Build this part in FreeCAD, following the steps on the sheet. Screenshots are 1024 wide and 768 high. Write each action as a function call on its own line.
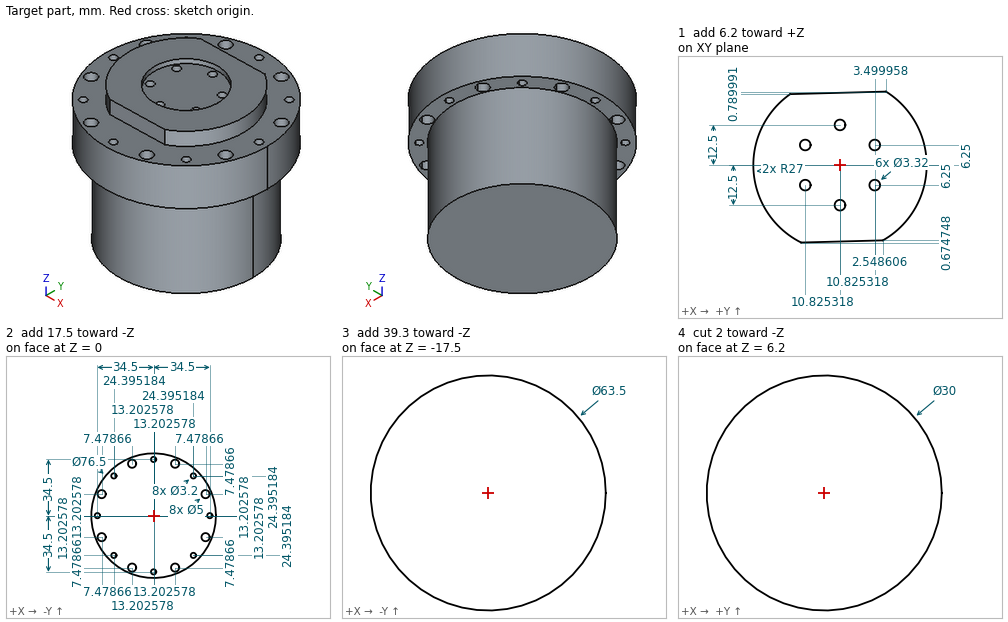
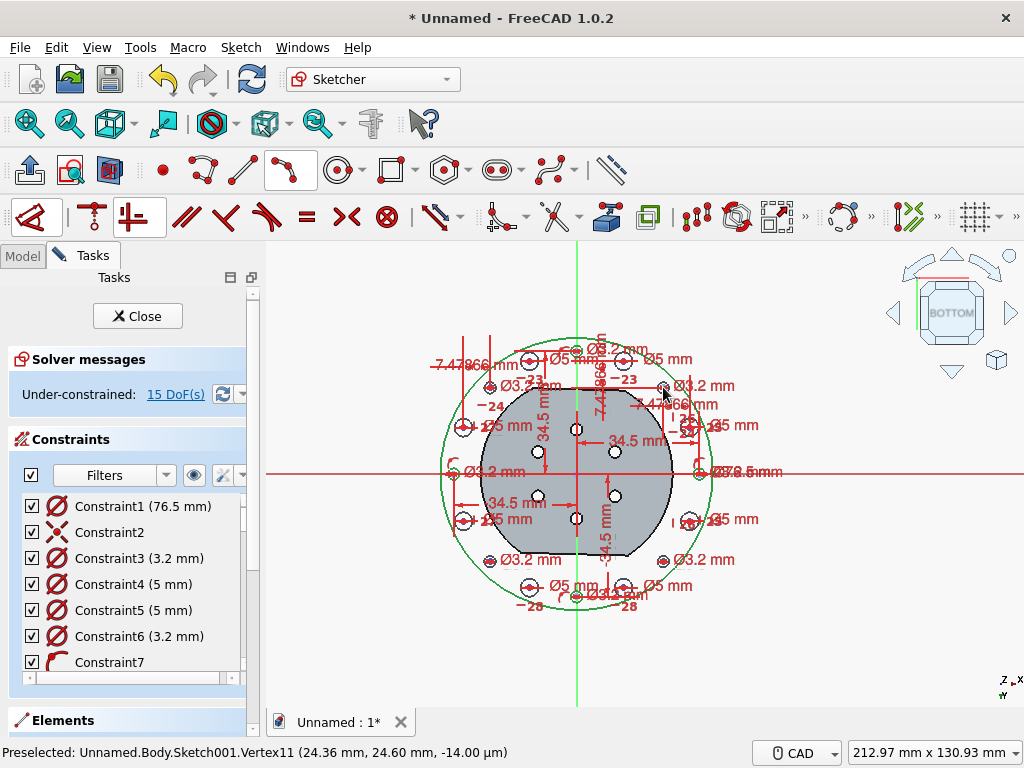
scroll(624, 588, up, 2)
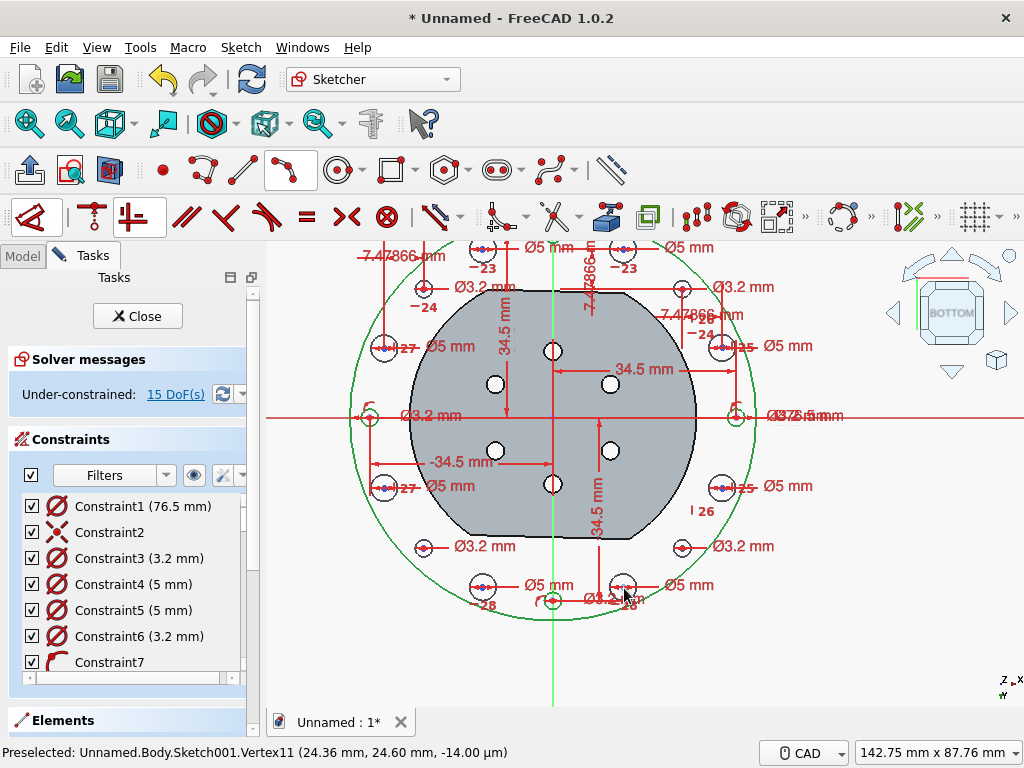
click(623, 587)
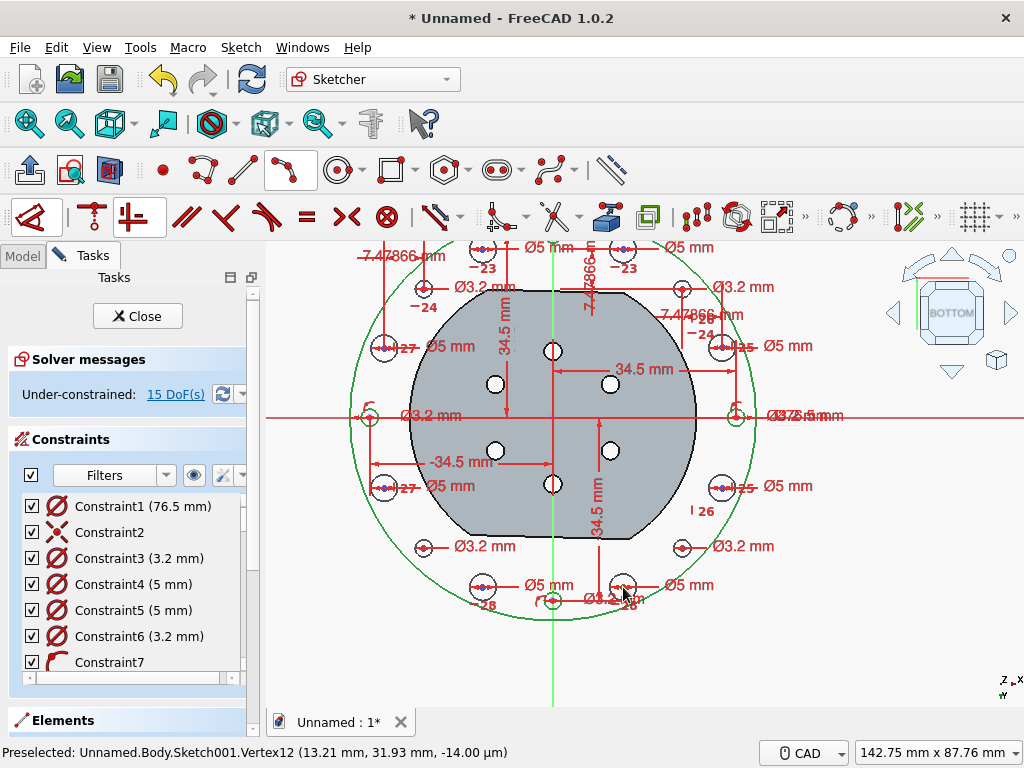
click(56, 218)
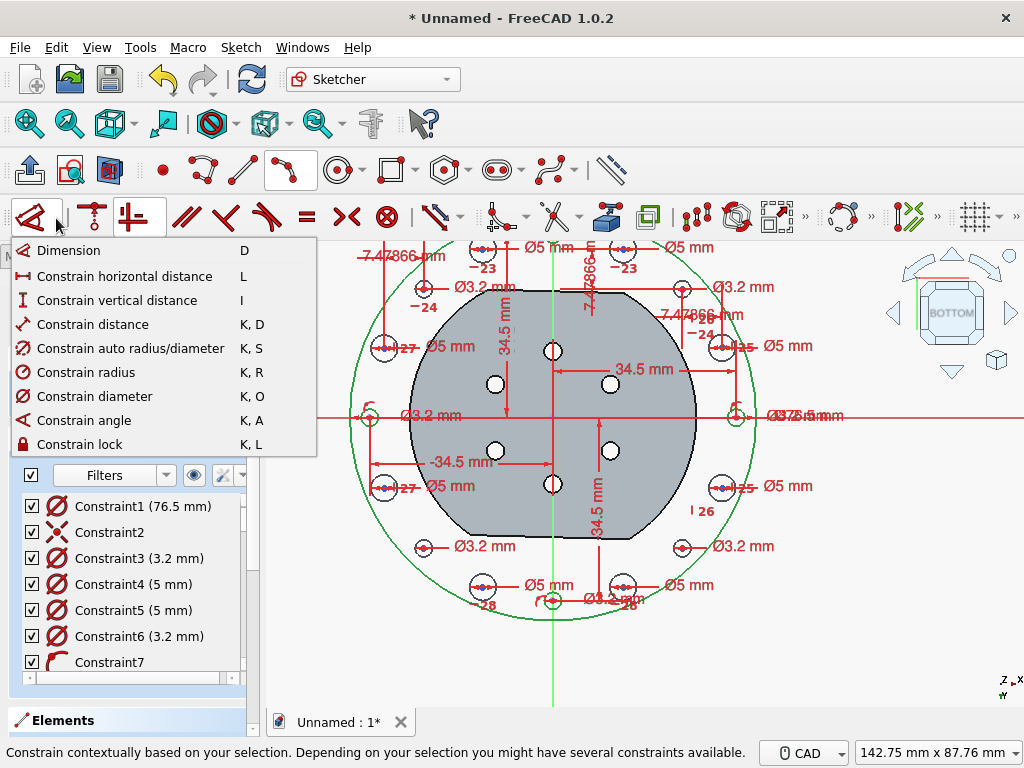
click(164, 300)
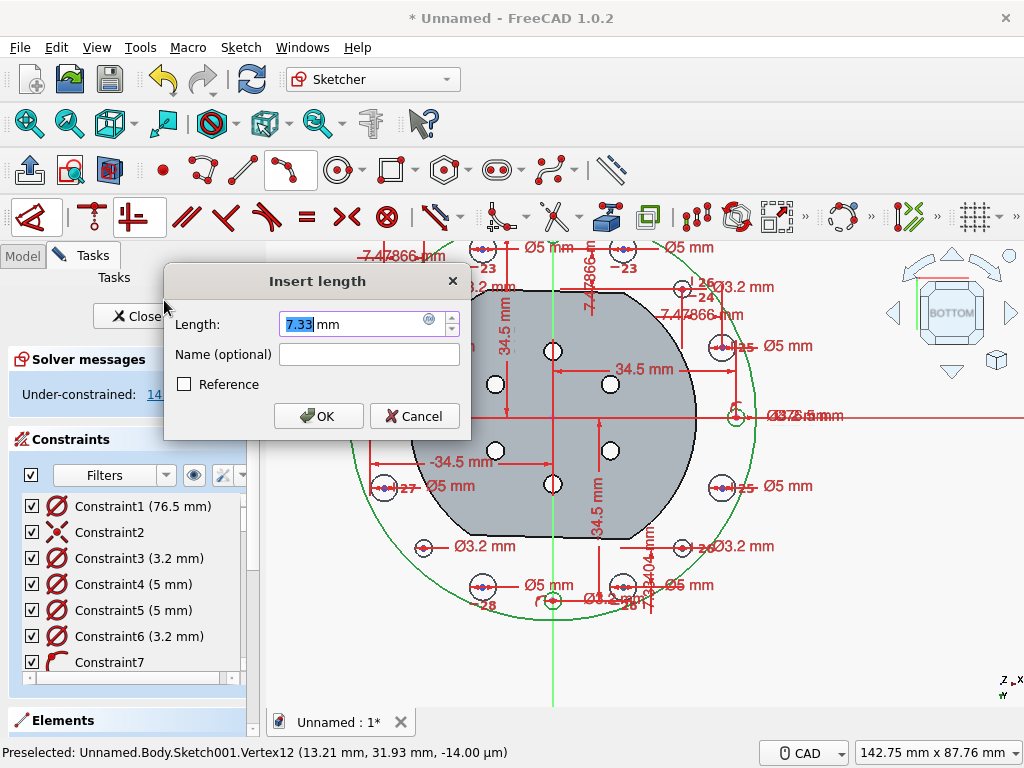
text(7.47866)
key(Return)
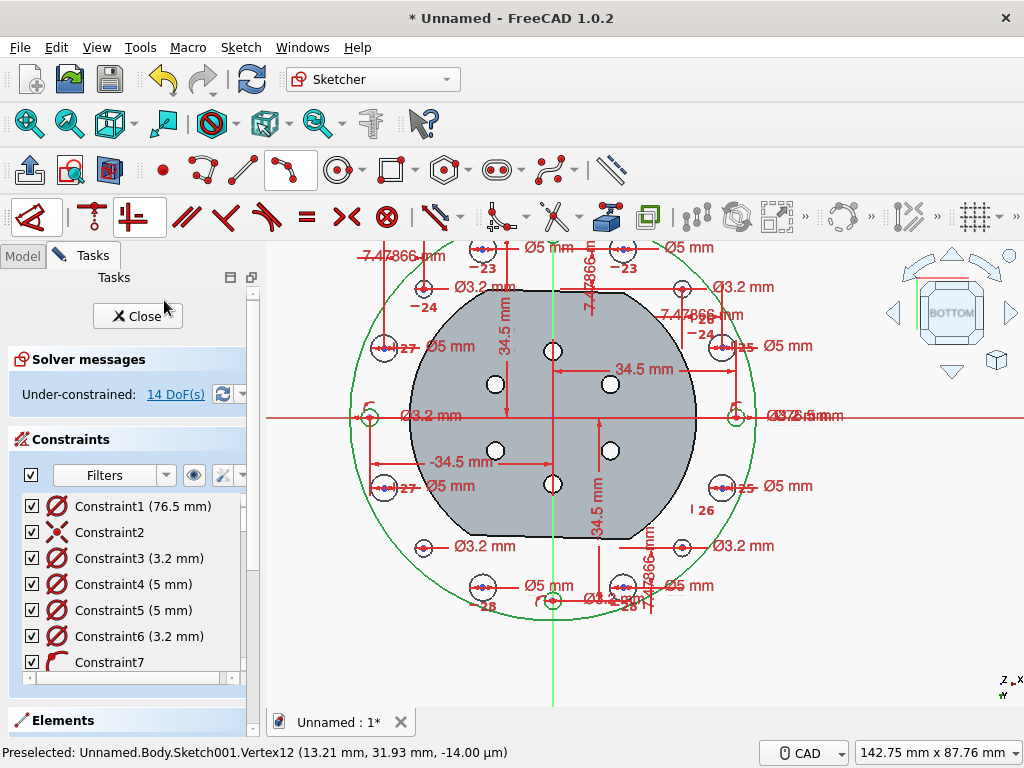
click(384, 488)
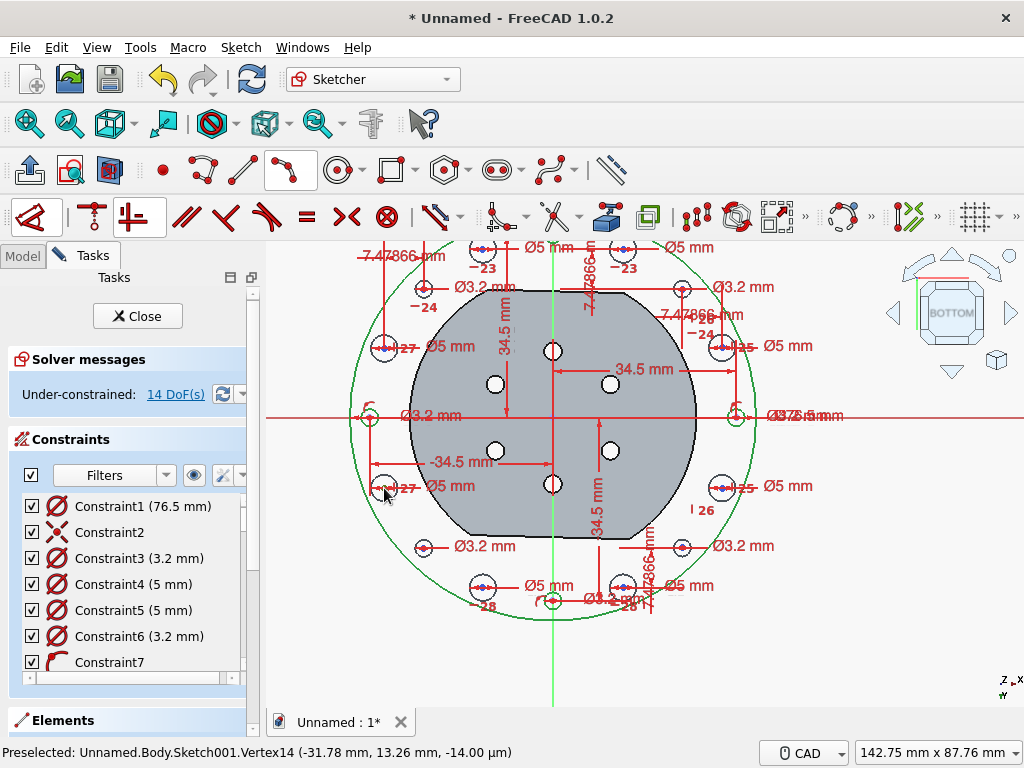
click(424, 548)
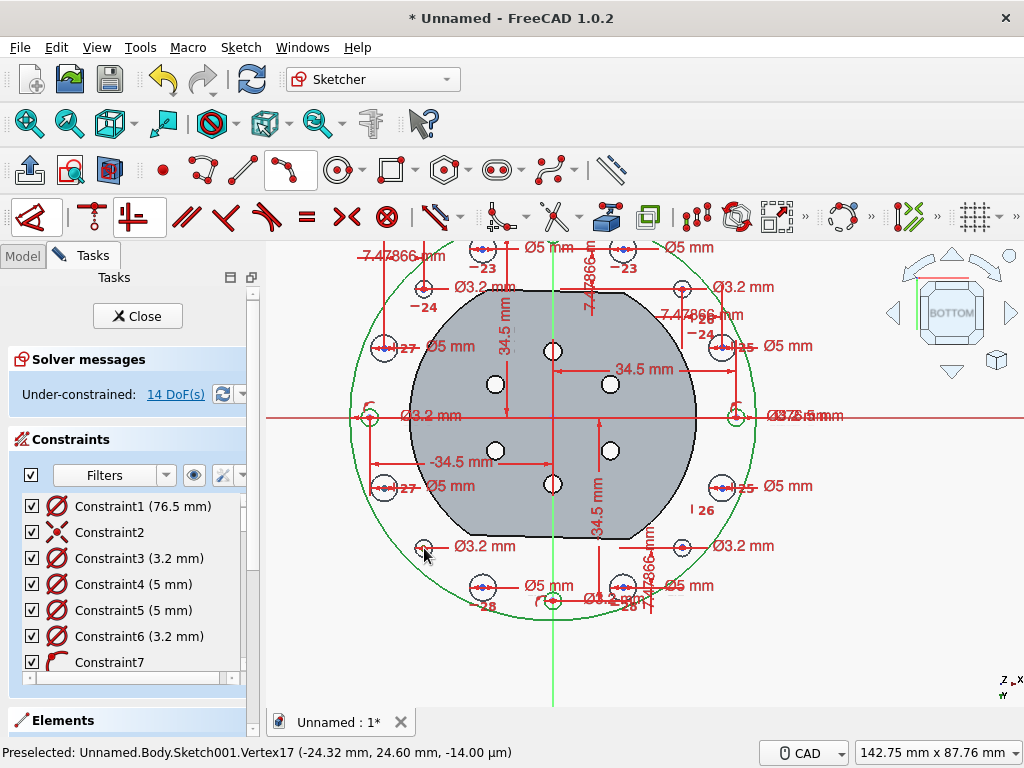
click(56, 218)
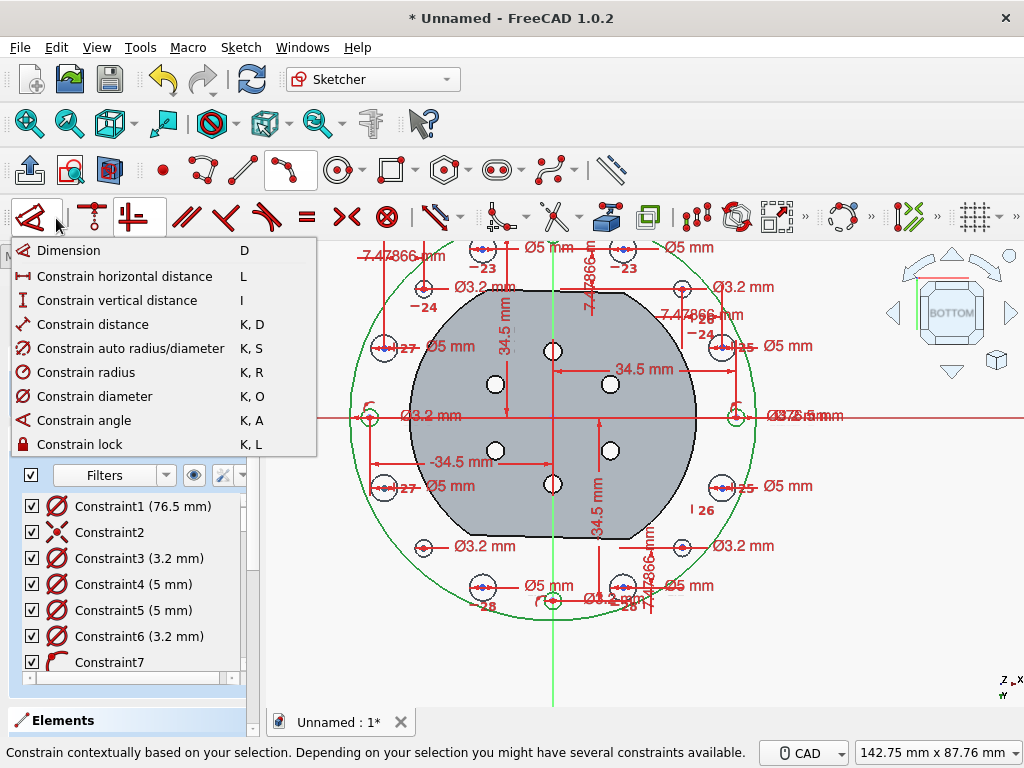
click(164, 276)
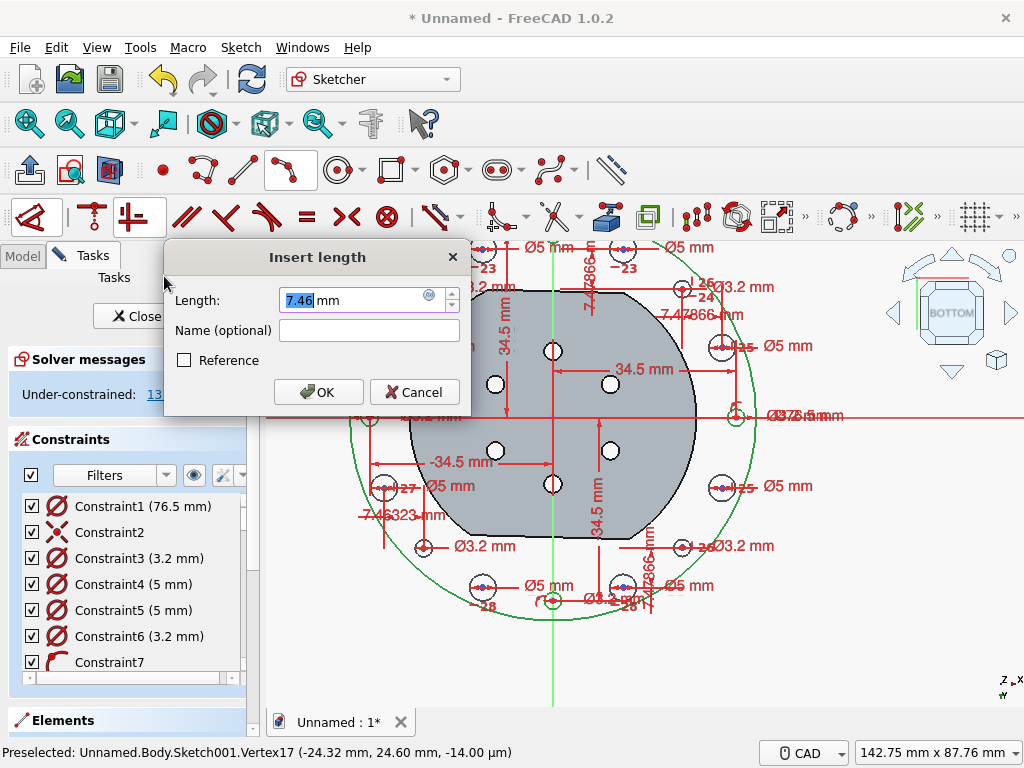
text(7.47866)
key(Return)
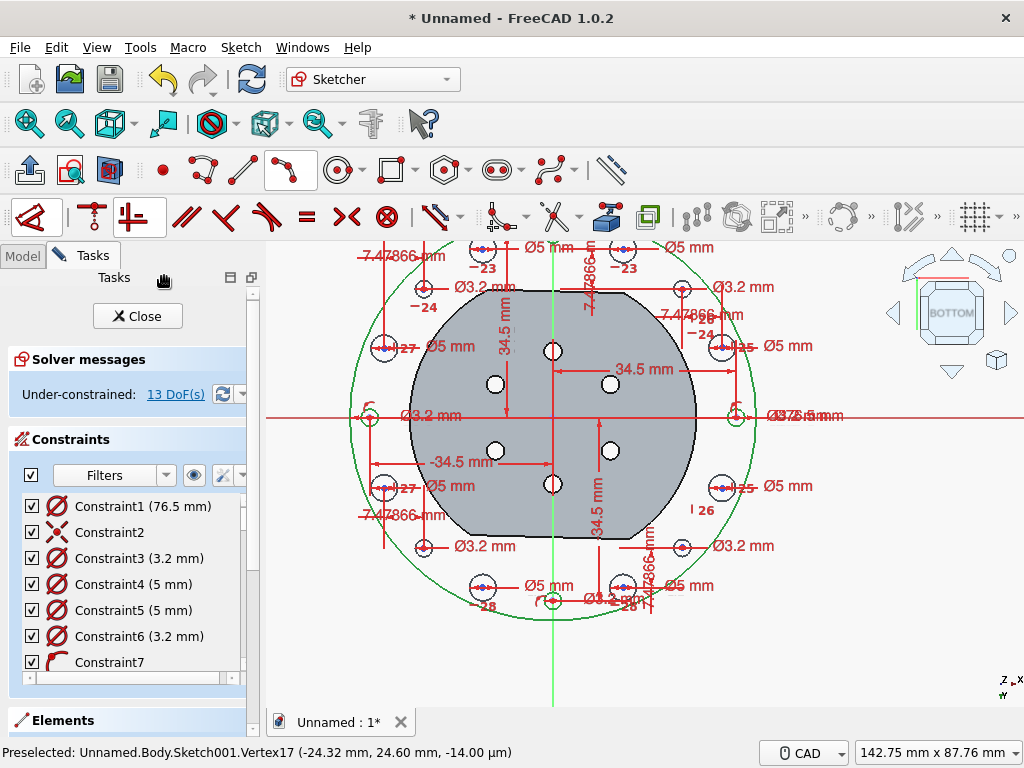
click(483, 588)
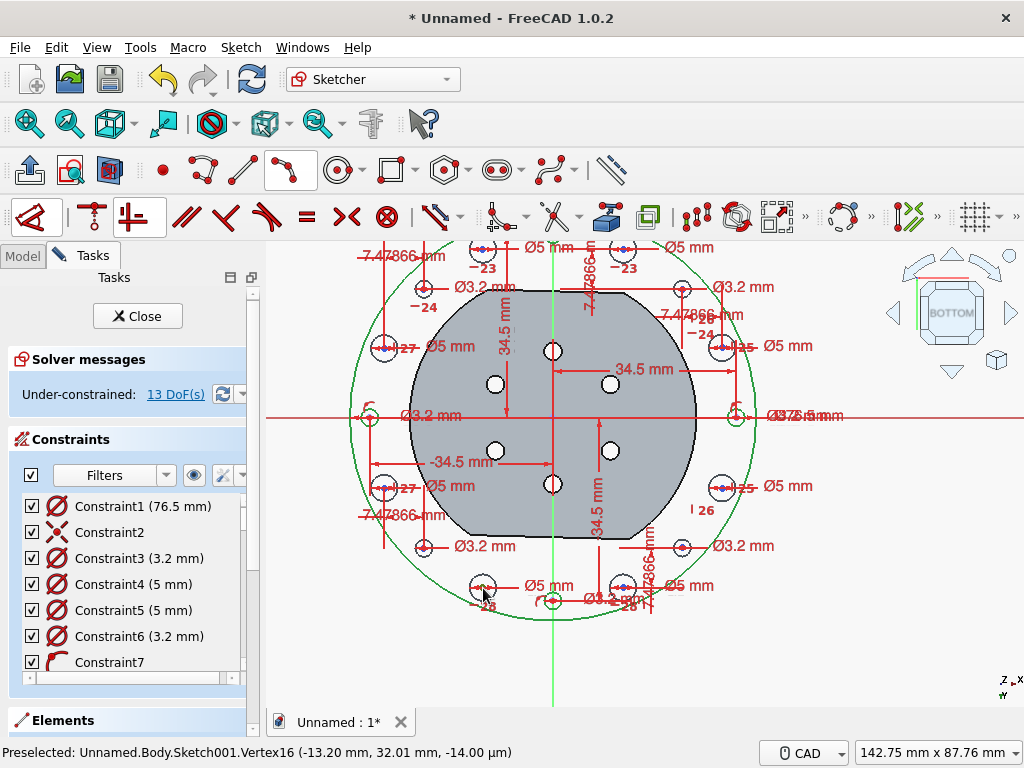
click(424, 548)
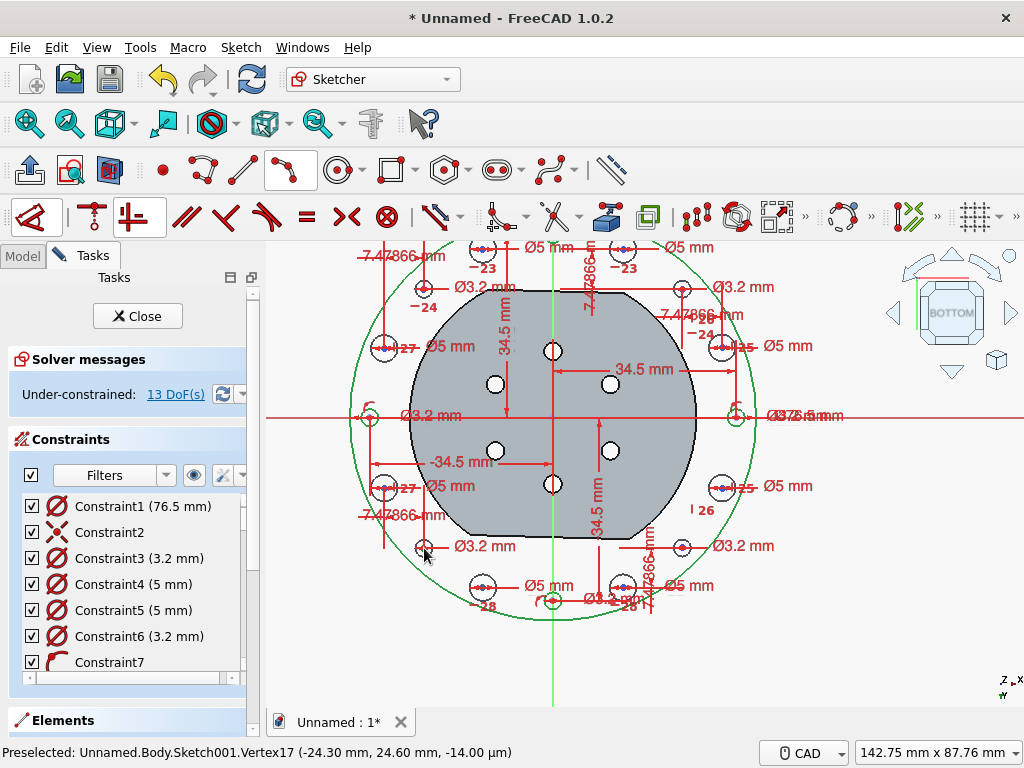
click(56, 218)